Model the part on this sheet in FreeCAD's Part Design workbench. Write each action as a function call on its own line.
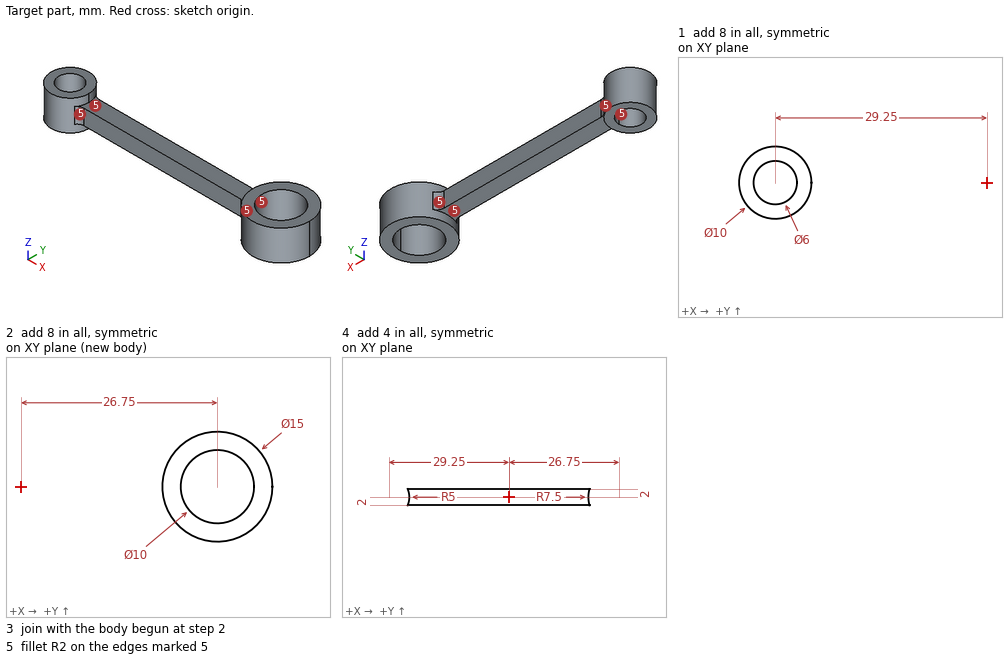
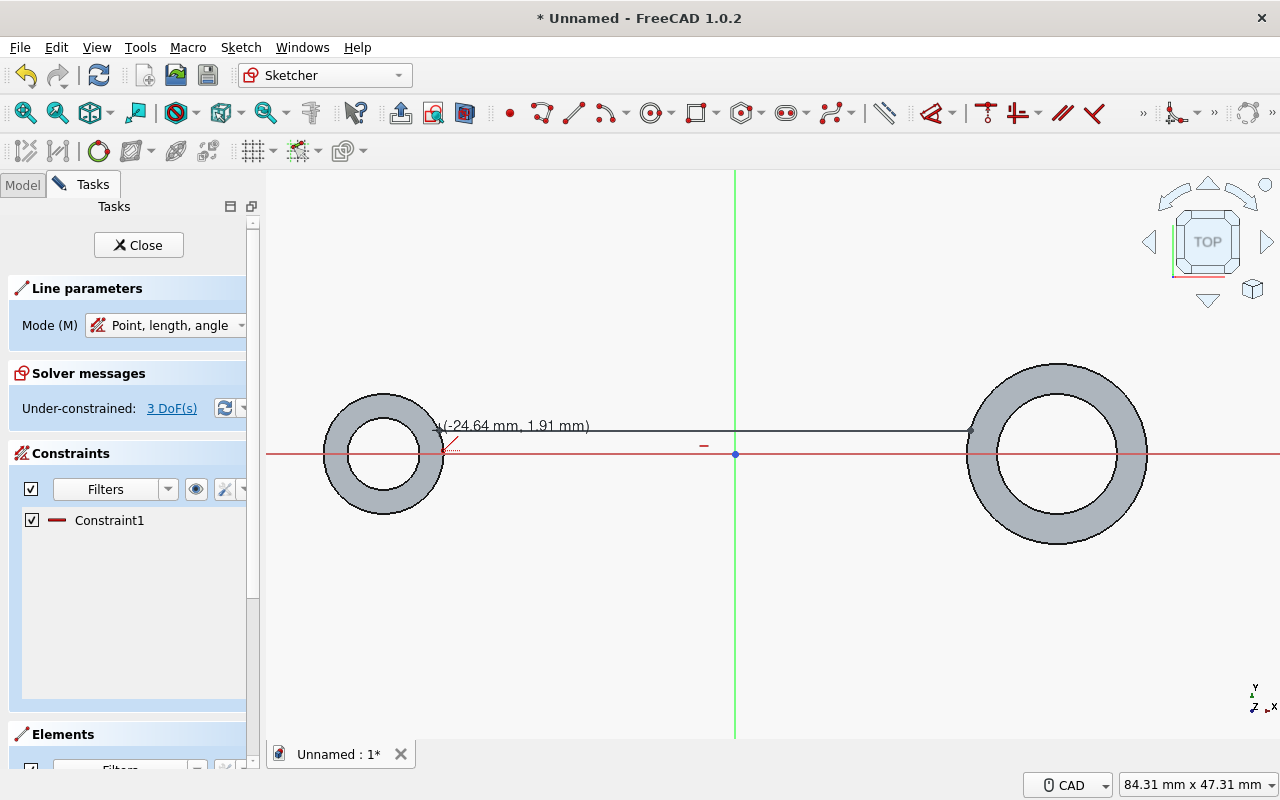
click(439, 478)
click(970, 478)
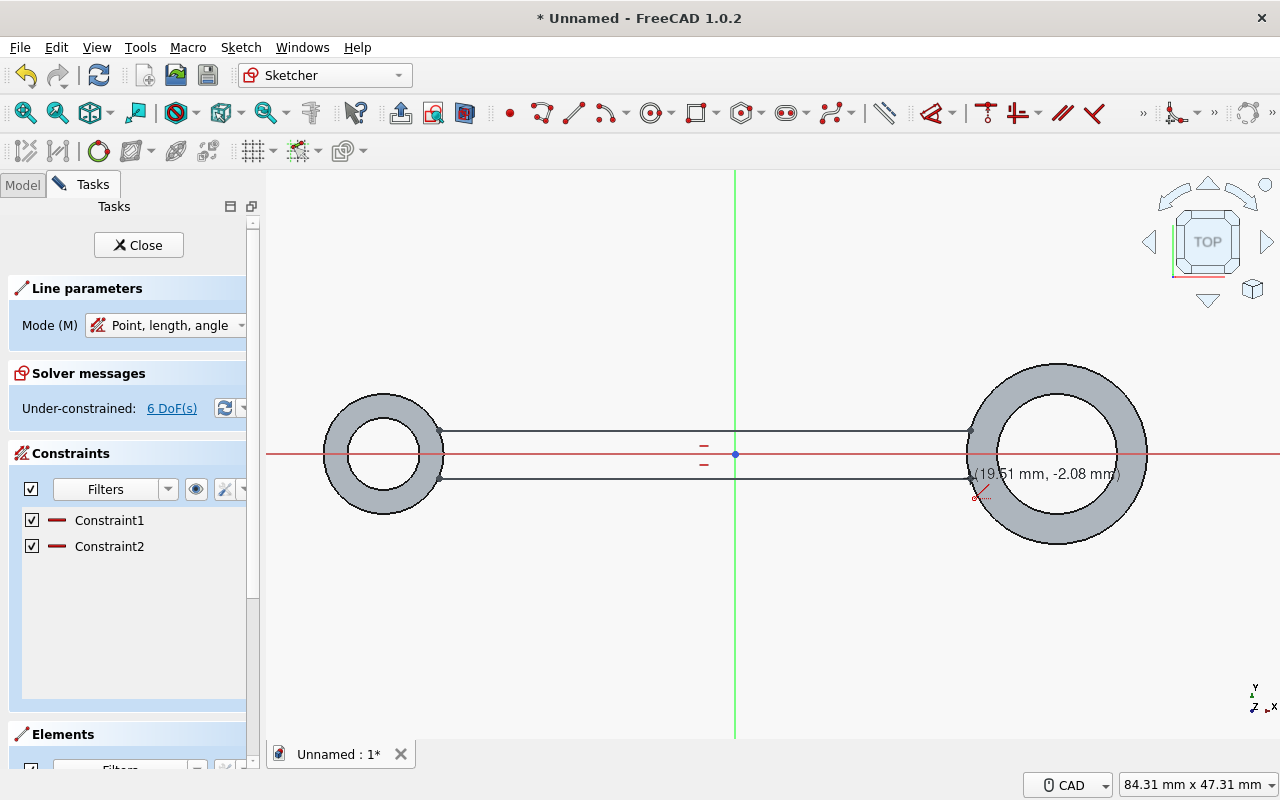
click(628, 114)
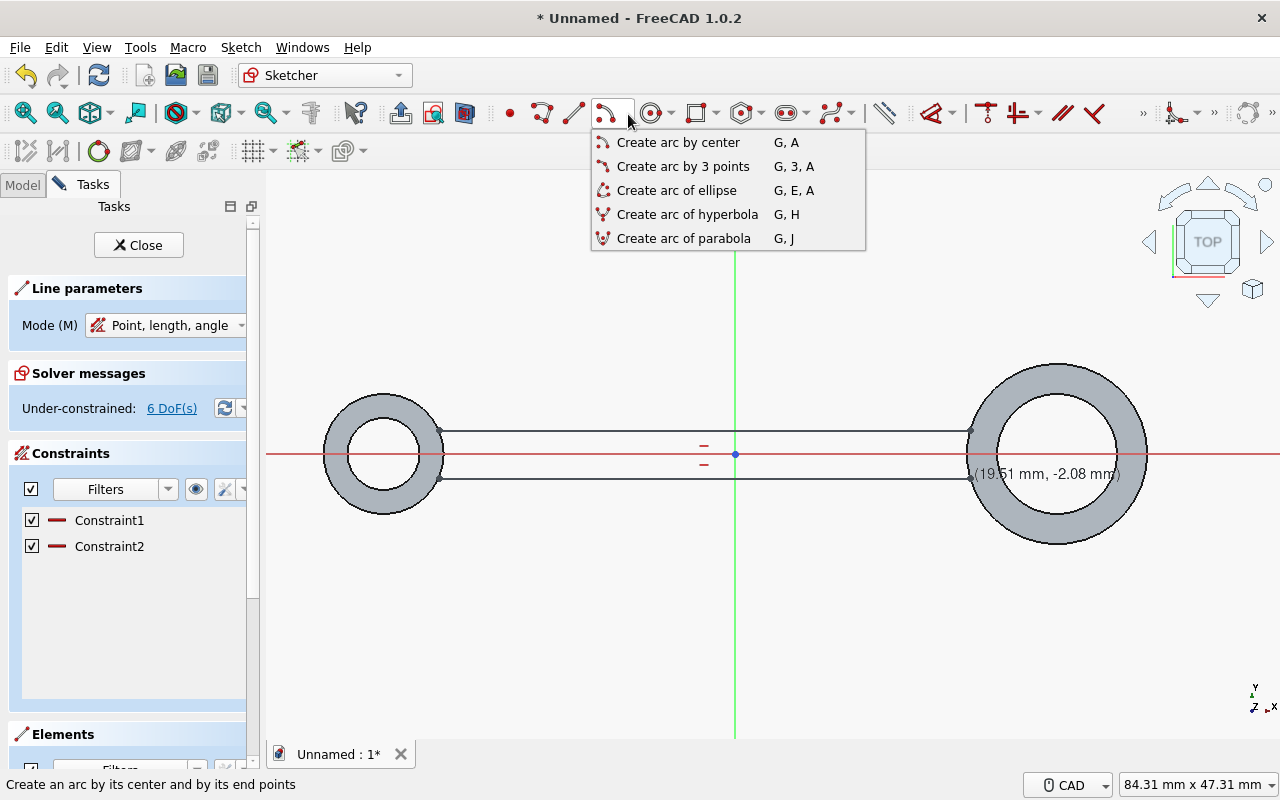
click(728, 166)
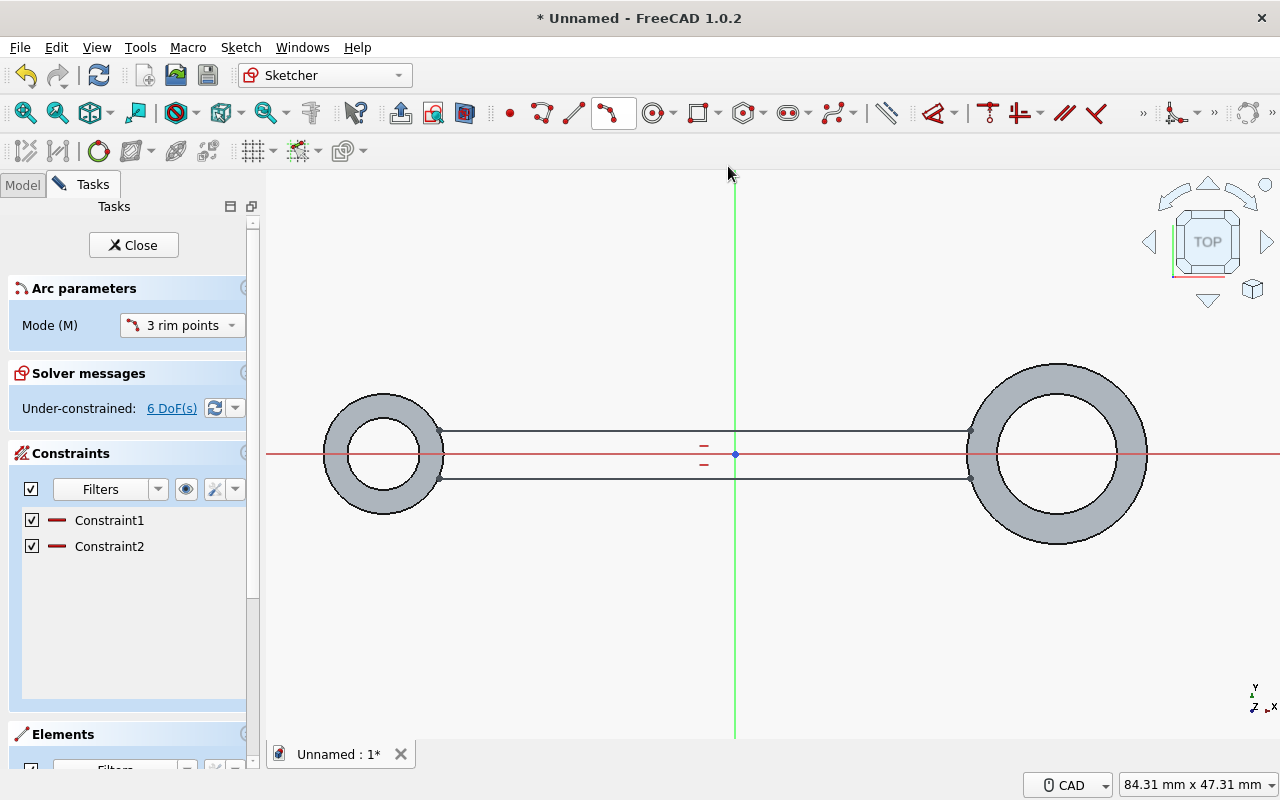
click(439, 431)
click(439, 479)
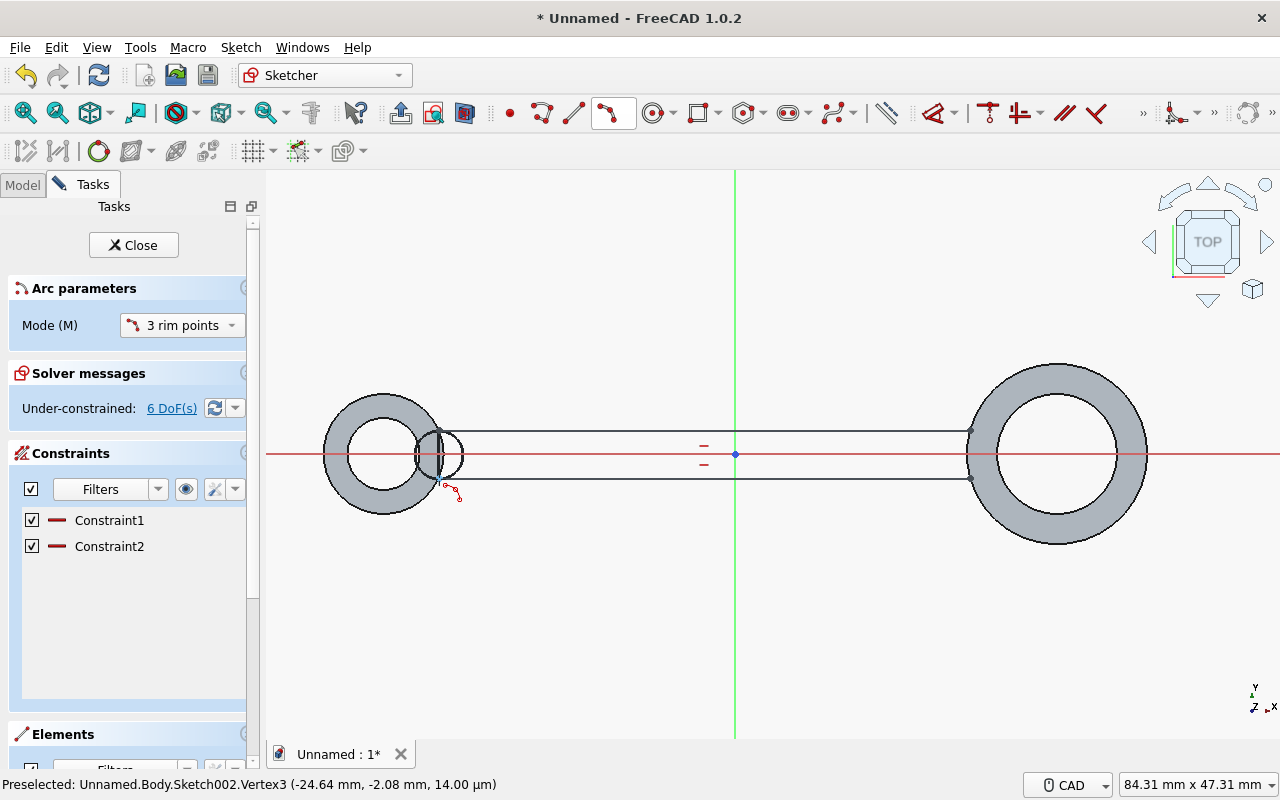
scroll(443, 459, up, 6)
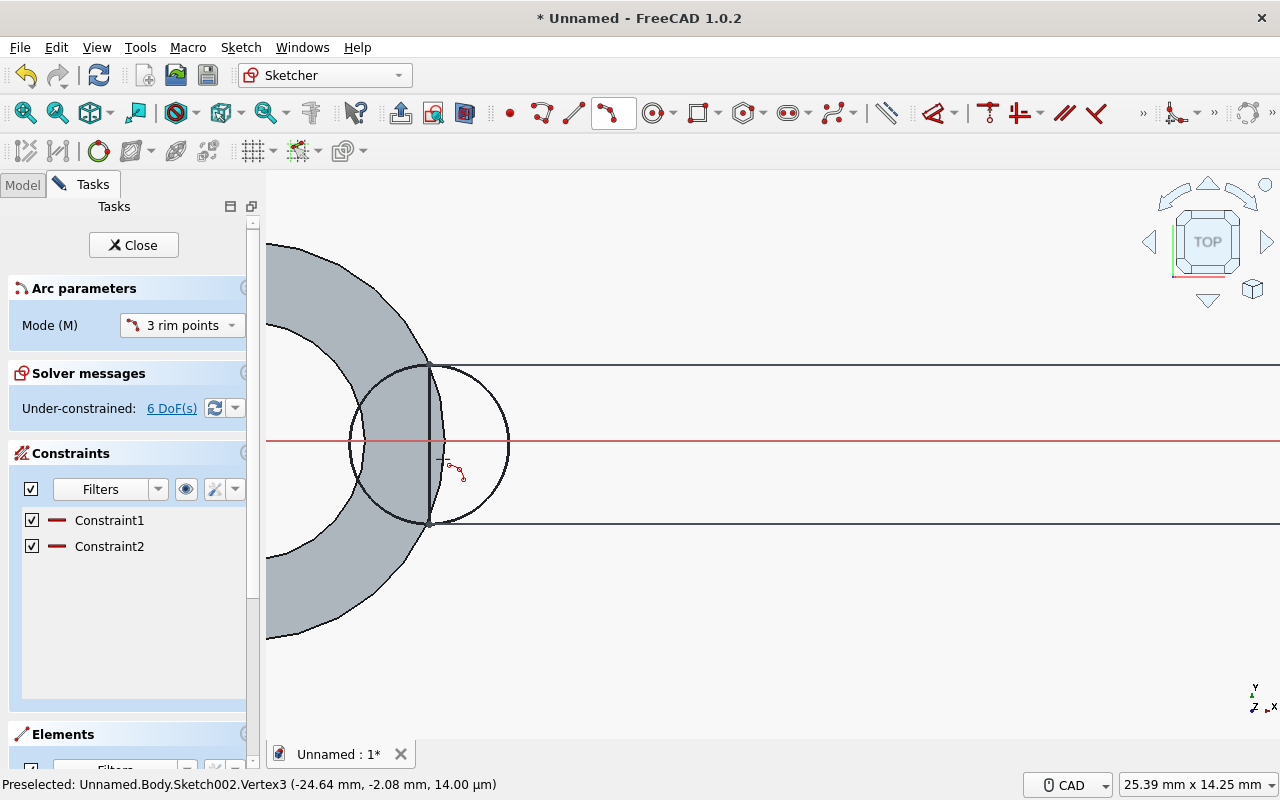
click(444, 458)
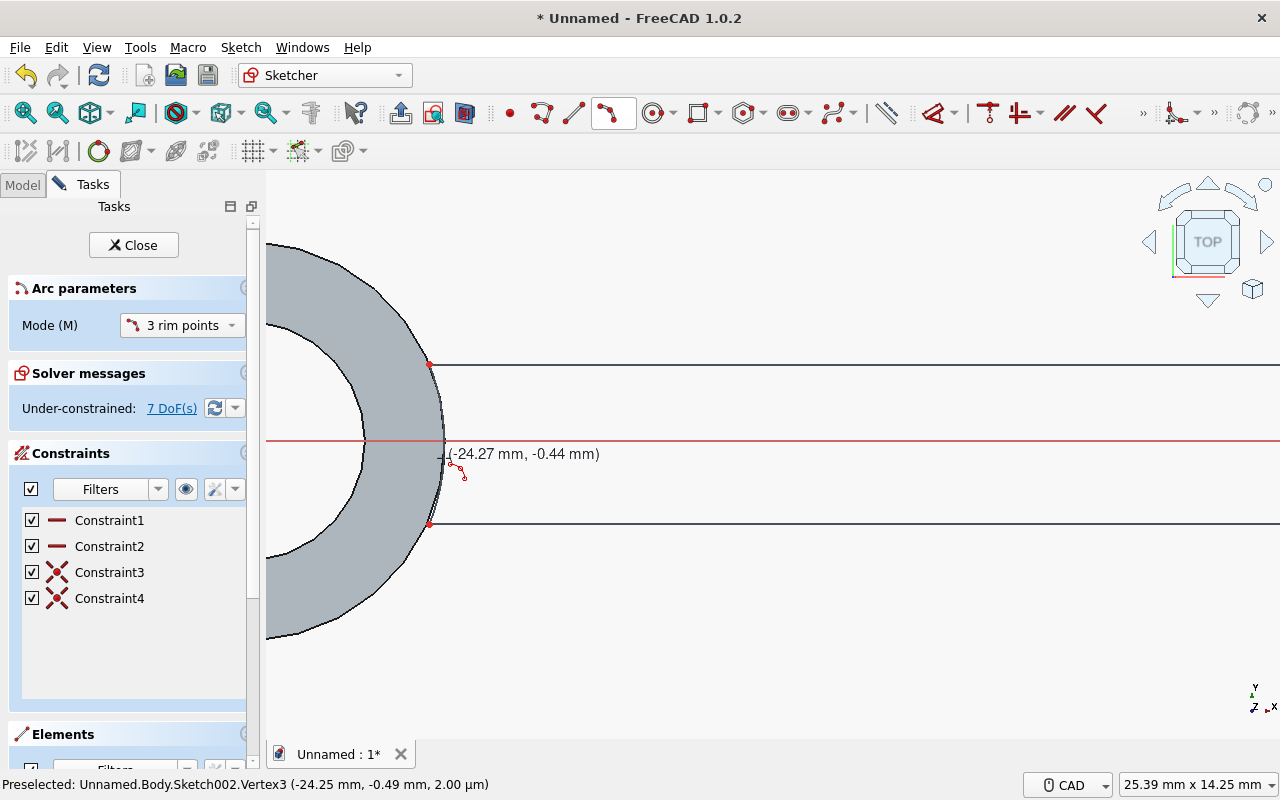
scroll(443, 460, down, 6)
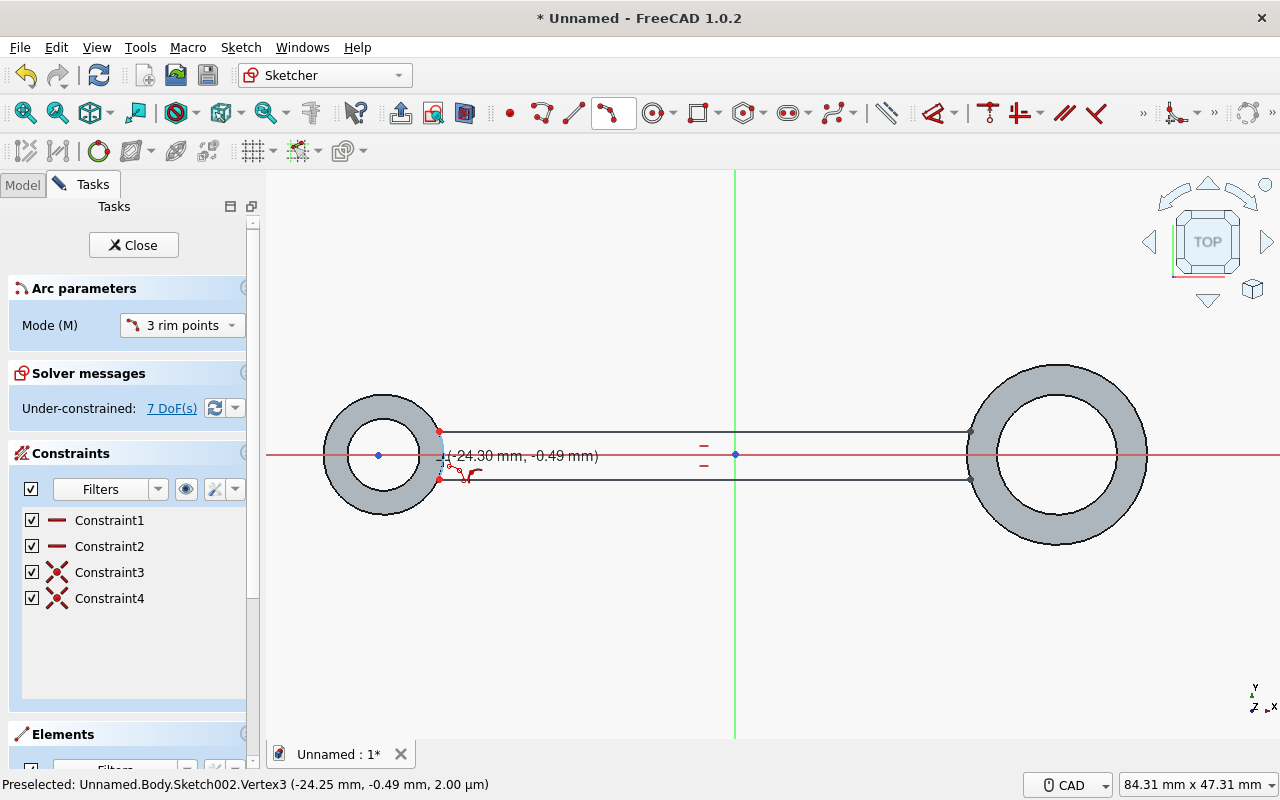
click(970, 480)
click(970, 432)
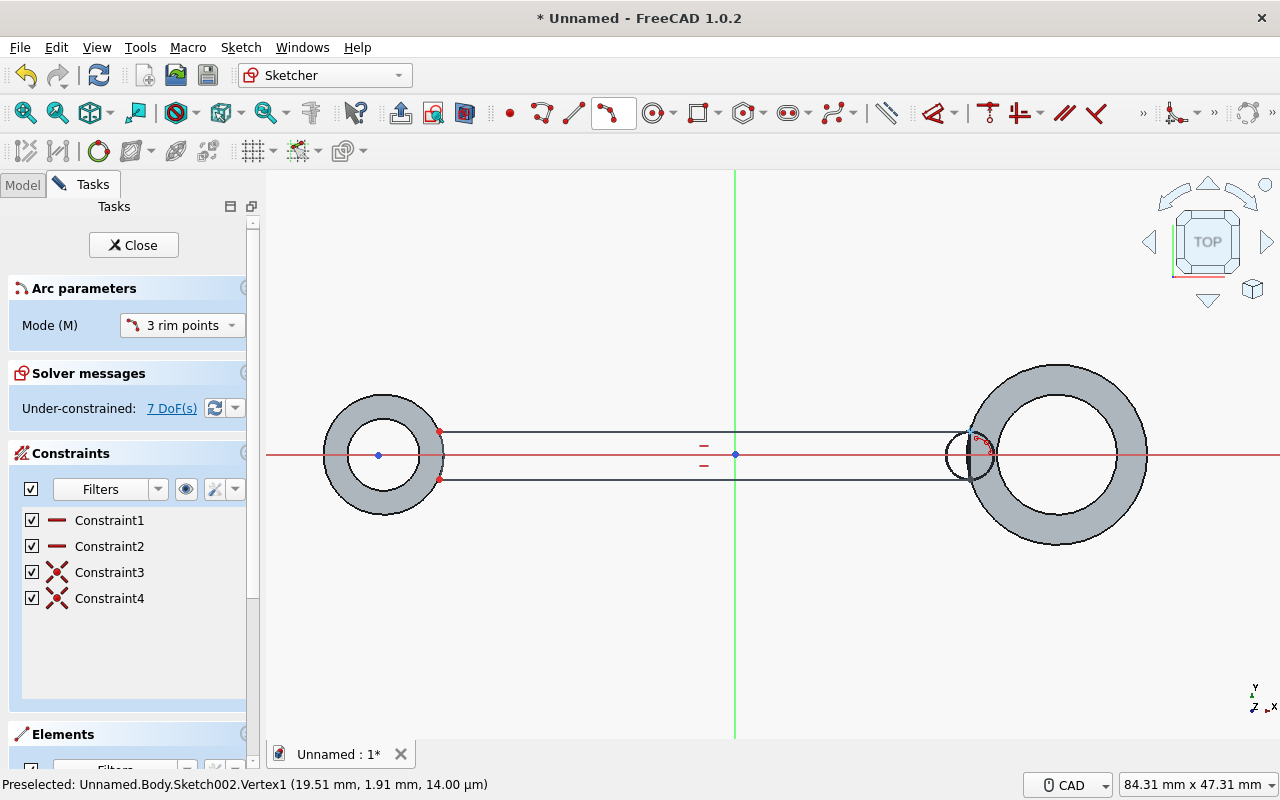
scroll(967, 450, up, 9)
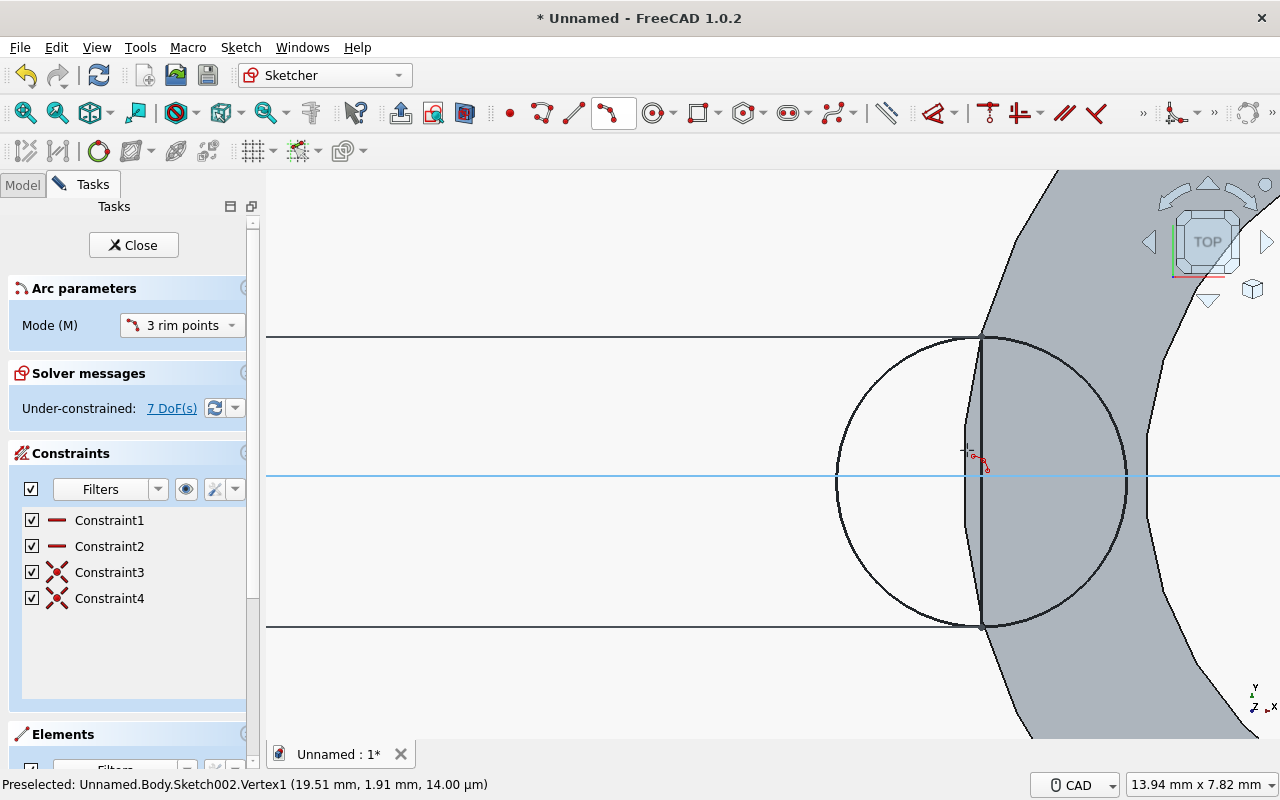
click(963, 447)
key(Escape)